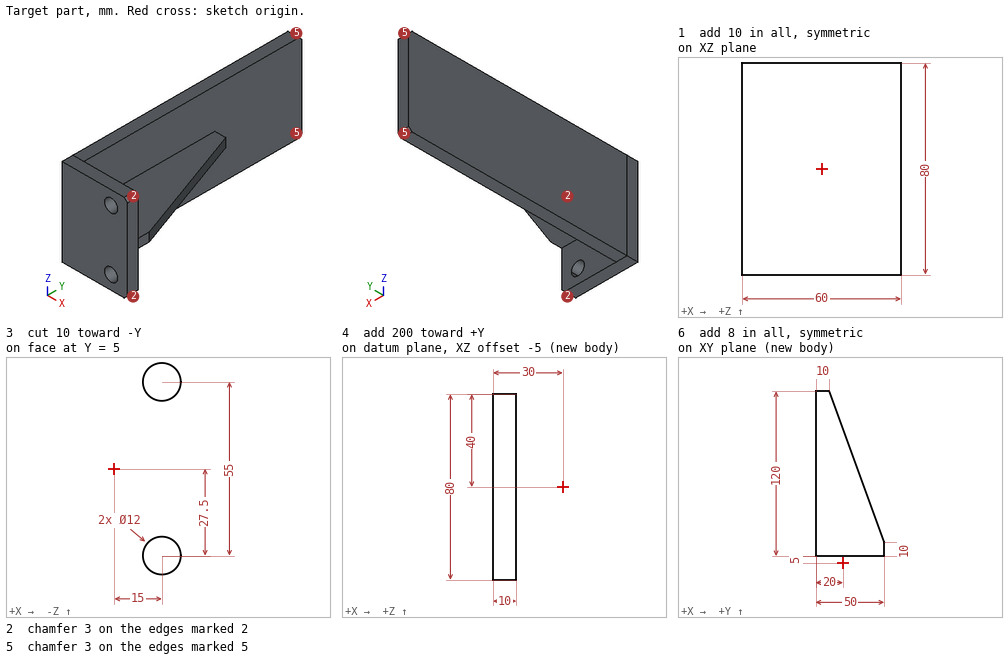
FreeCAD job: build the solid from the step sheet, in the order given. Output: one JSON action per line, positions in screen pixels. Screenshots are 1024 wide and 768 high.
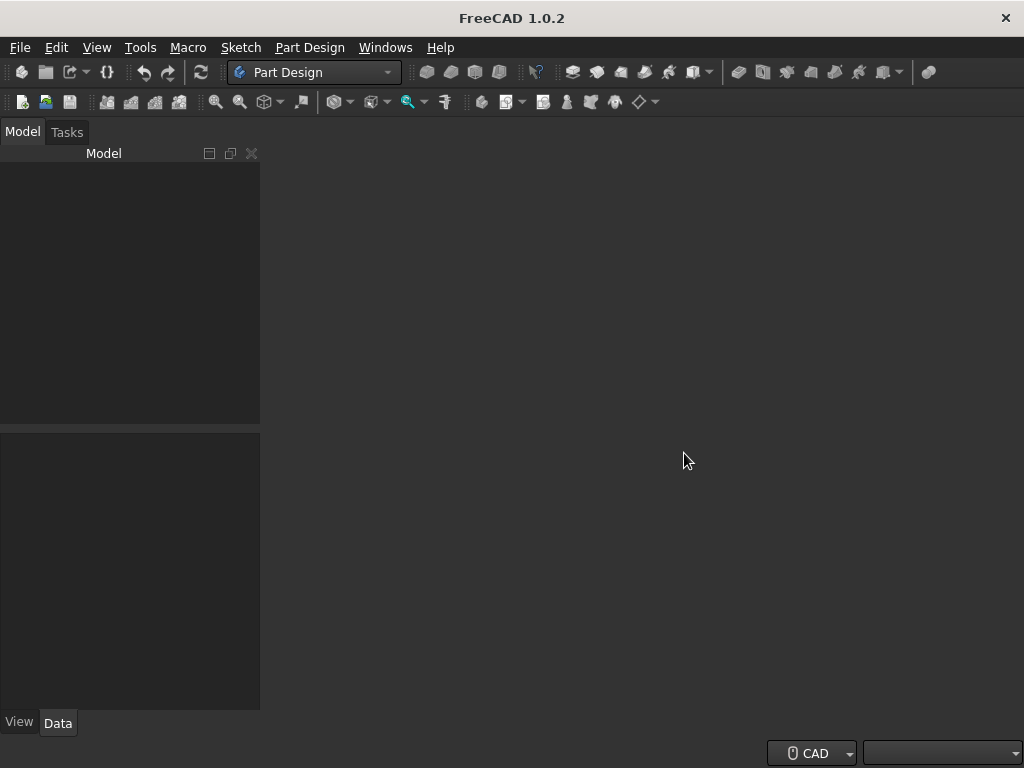
{"action": "left_click", "coordinate": [22, 102]}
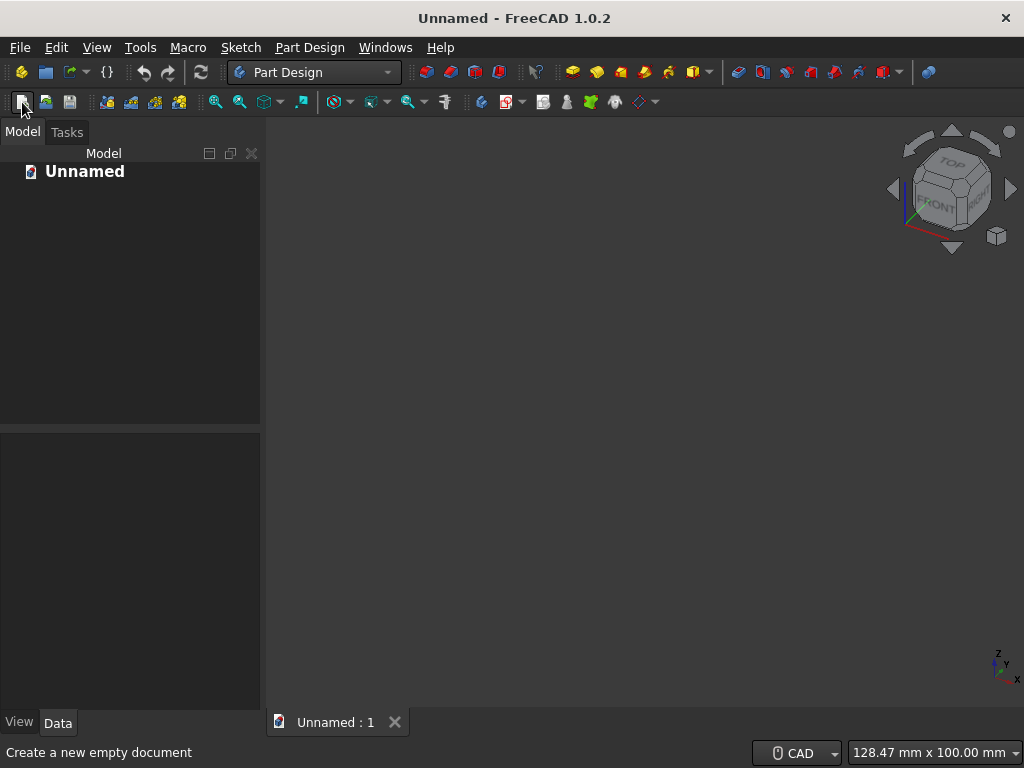
{"action": "left_click", "coordinate": [506, 102]}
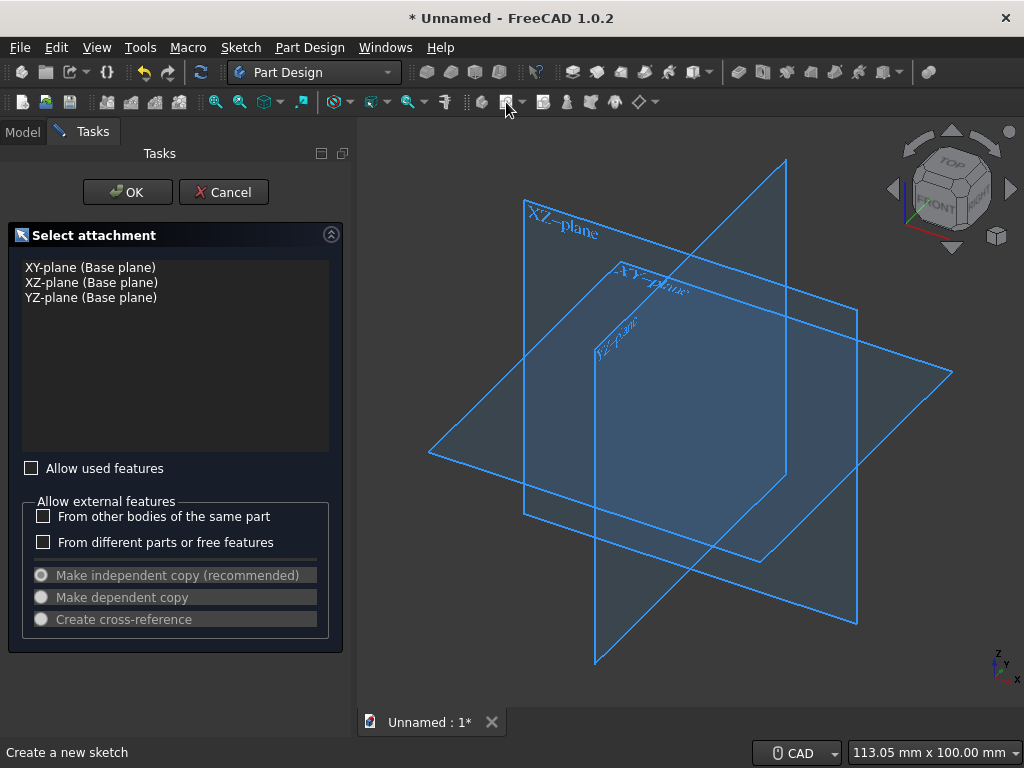
{"action": "left_click", "coordinate": [82, 282]}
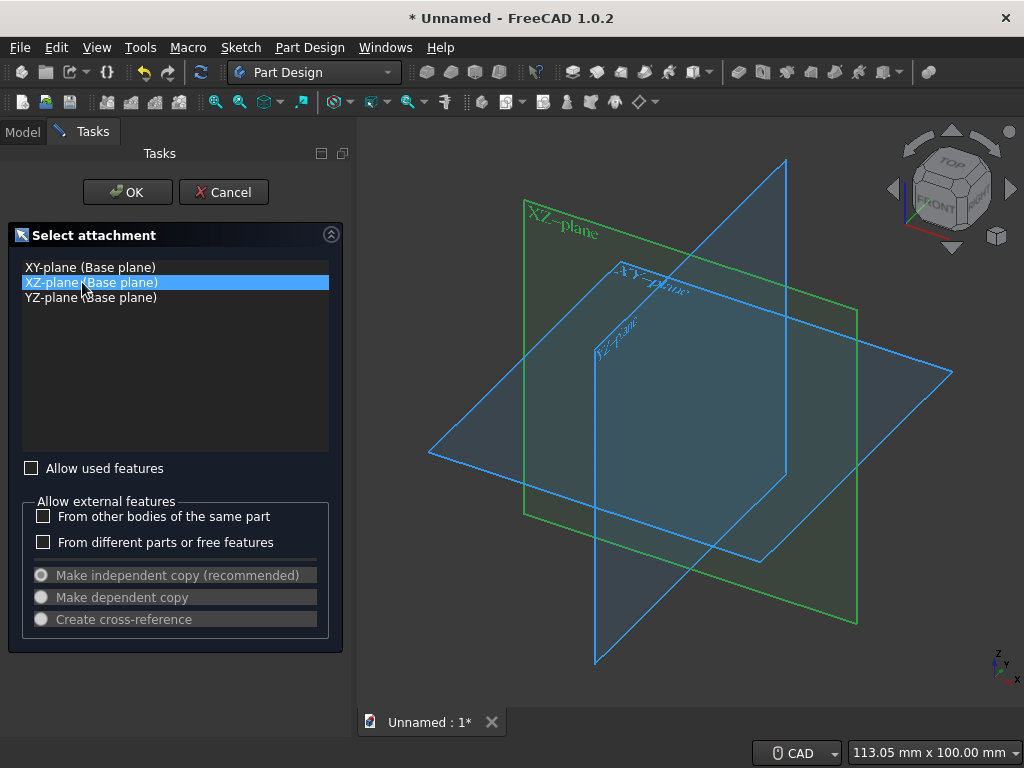
{"action": "left_click", "coordinate": [128, 192]}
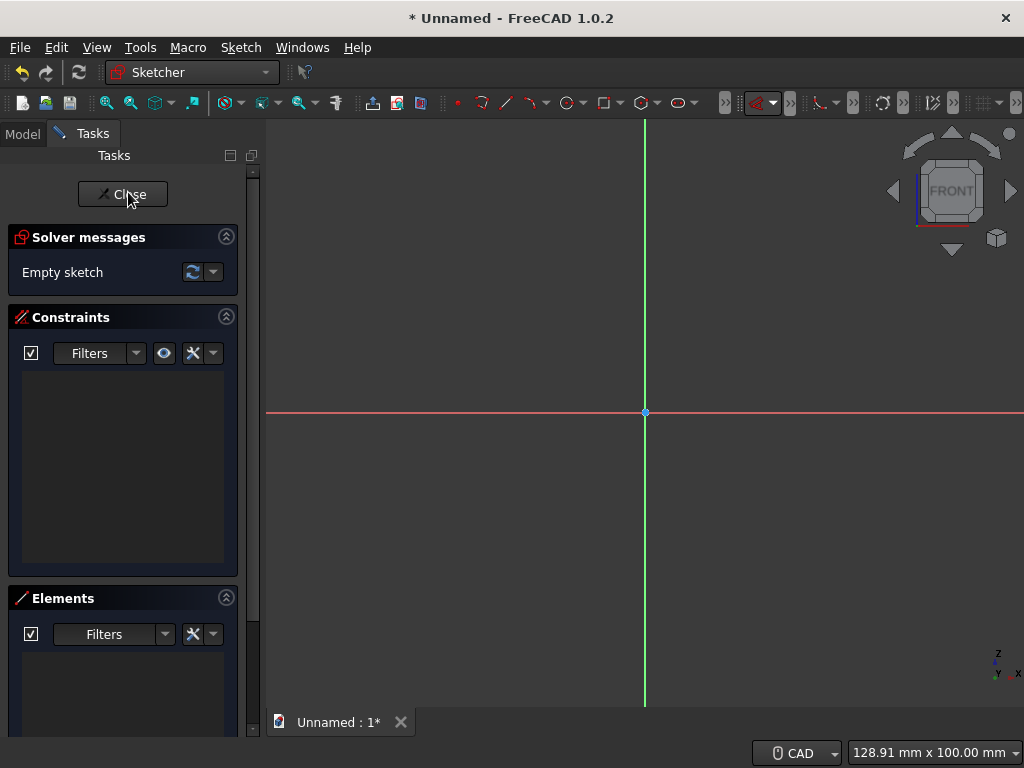
{"action": "key", "text": "g v"}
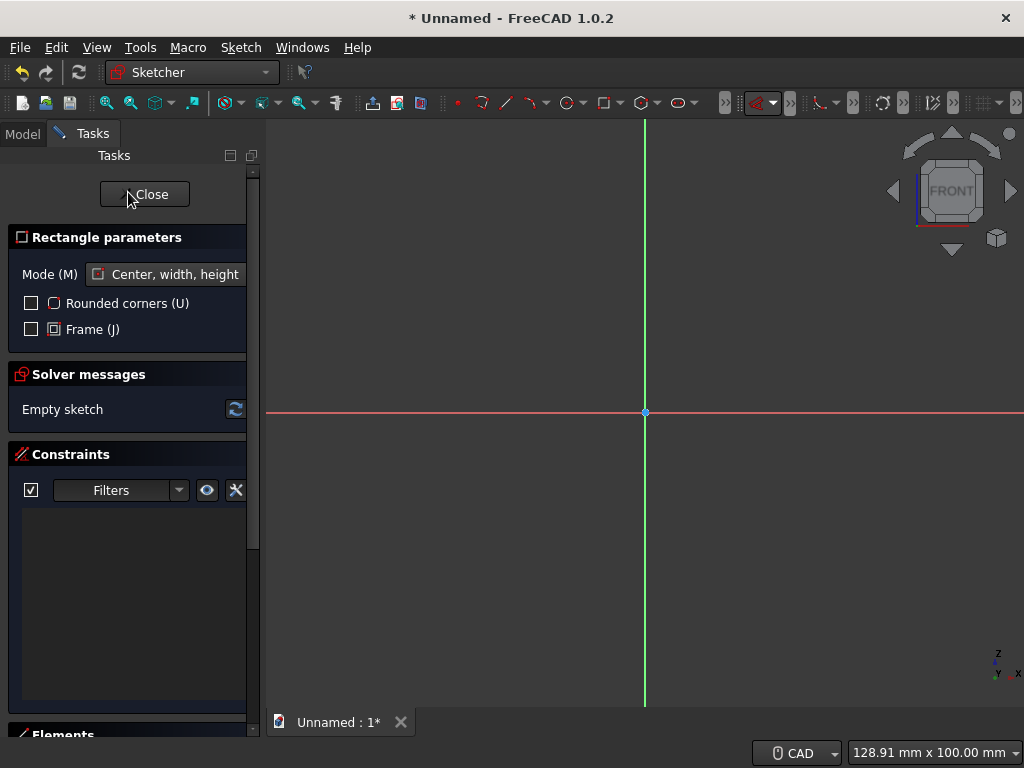
{"action": "left_click", "coordinate": [645, 413]}
{"action": "mouse_move", "coordinate": [821, 178]}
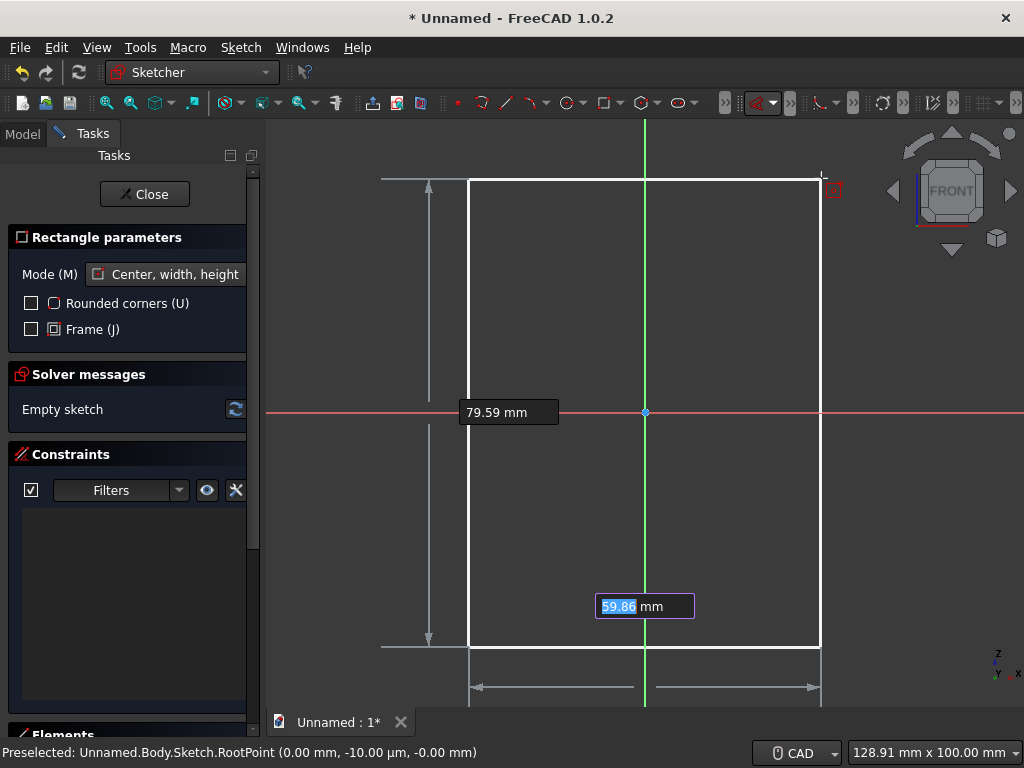
{"action": "type", "text": "60"}
{"action": "key", "text": "Tab"}
{"action": "type", "text": "80"}
{"action": "key", "text": "Return"}
{"action": "key", "text": "Escape"}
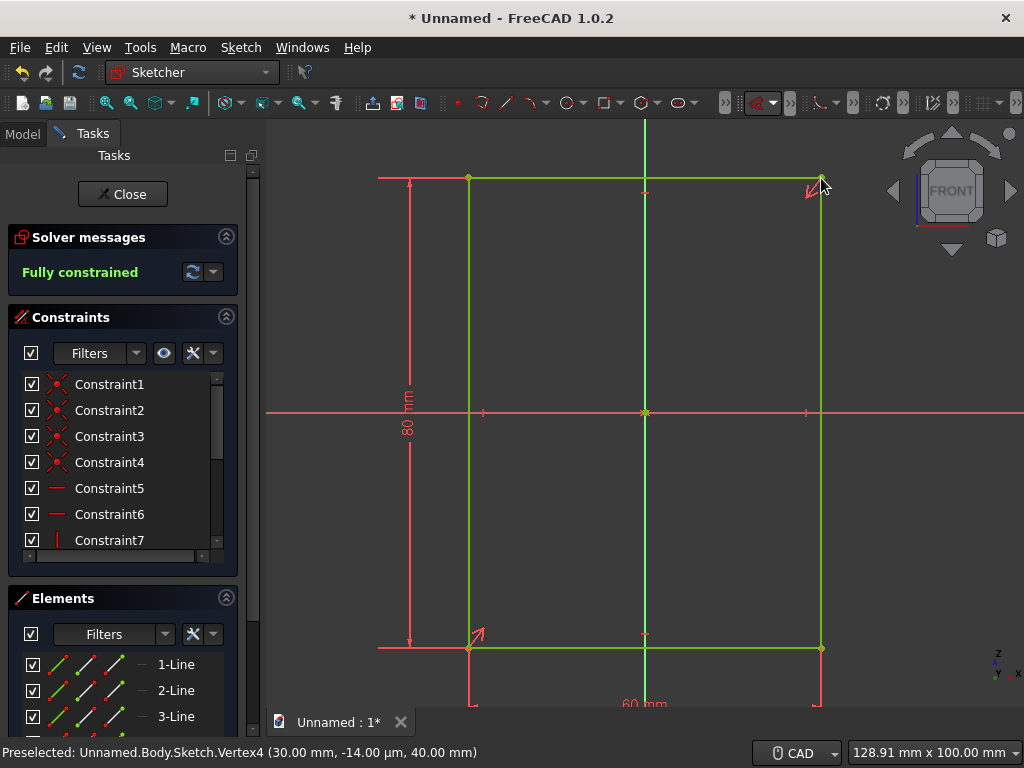
{"action": "left_click", "coordinate": [123, 194]}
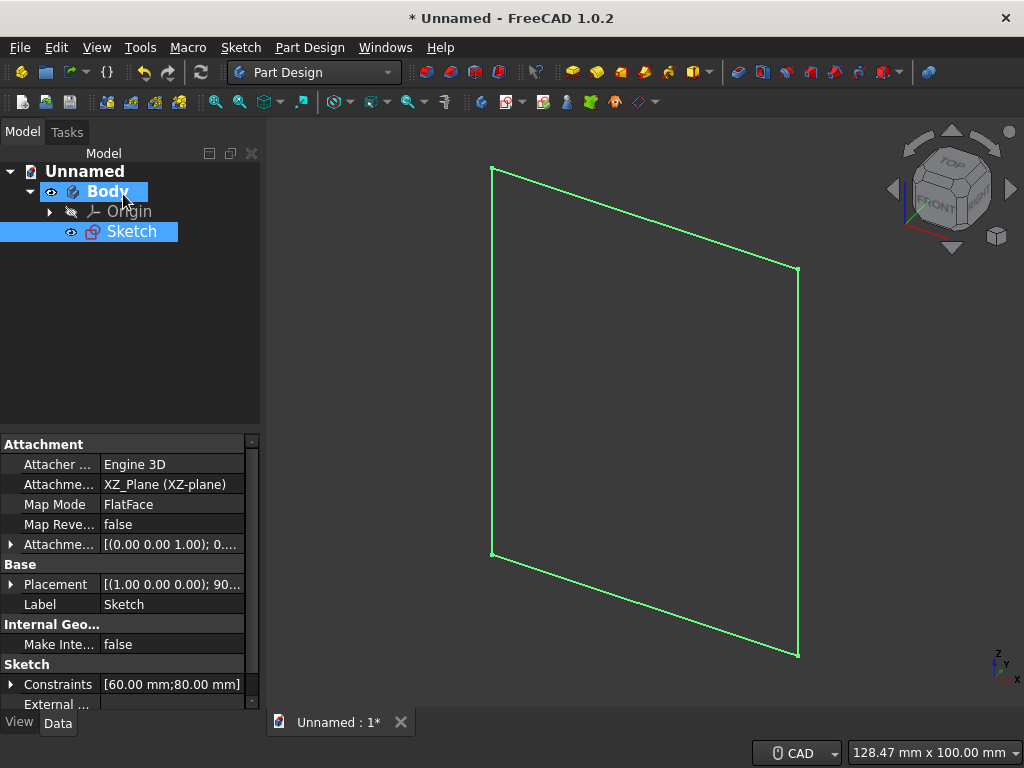
{"action": "left_click", "coordinate": [574, 72]}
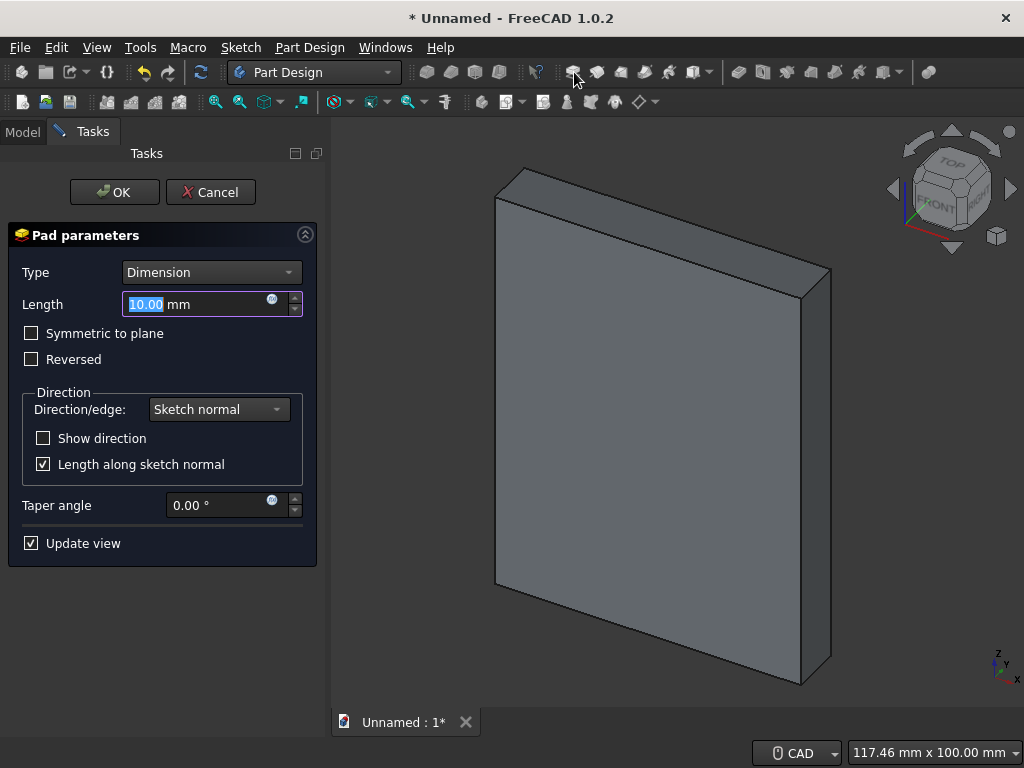
{"action": "type", "text": "10"}
{"action": "key", "text": "Tab"}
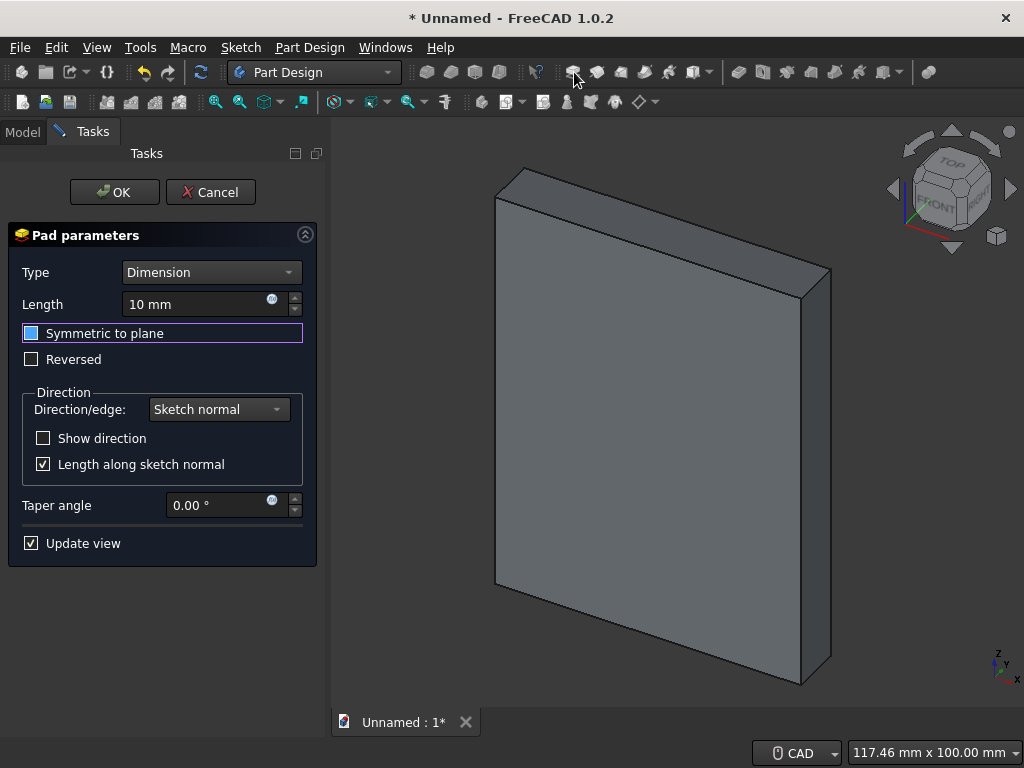
{"action": "left_click", "coordinate": [30, 333]}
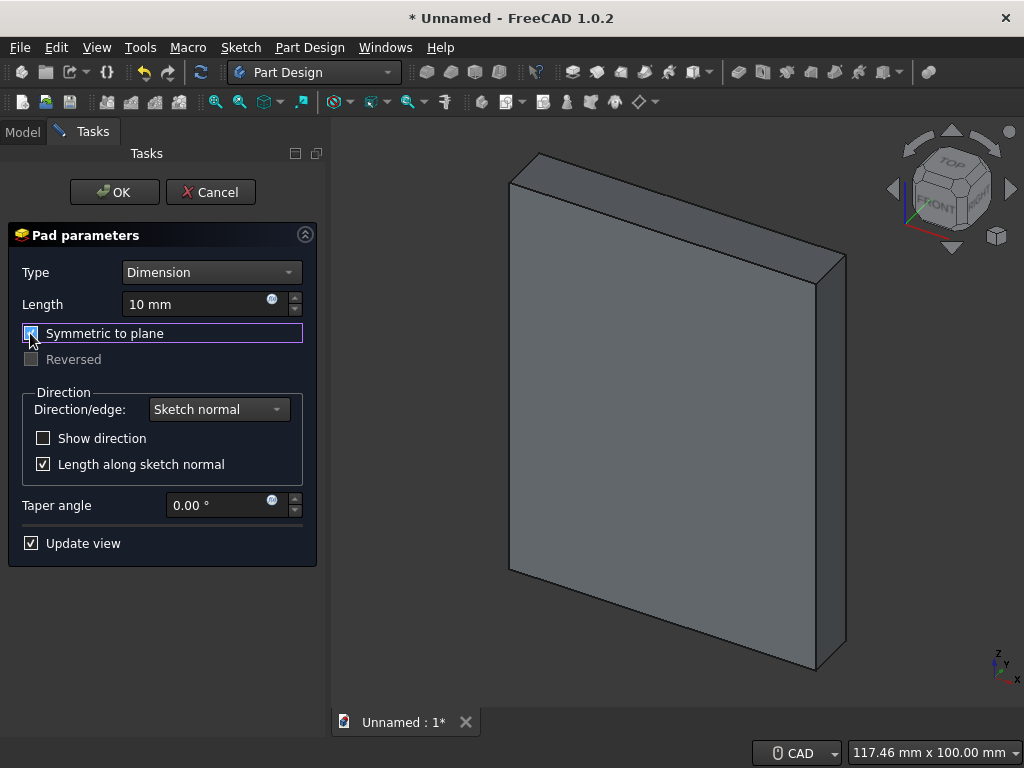
{"action": "left_click", "coordinate": [115, 192]}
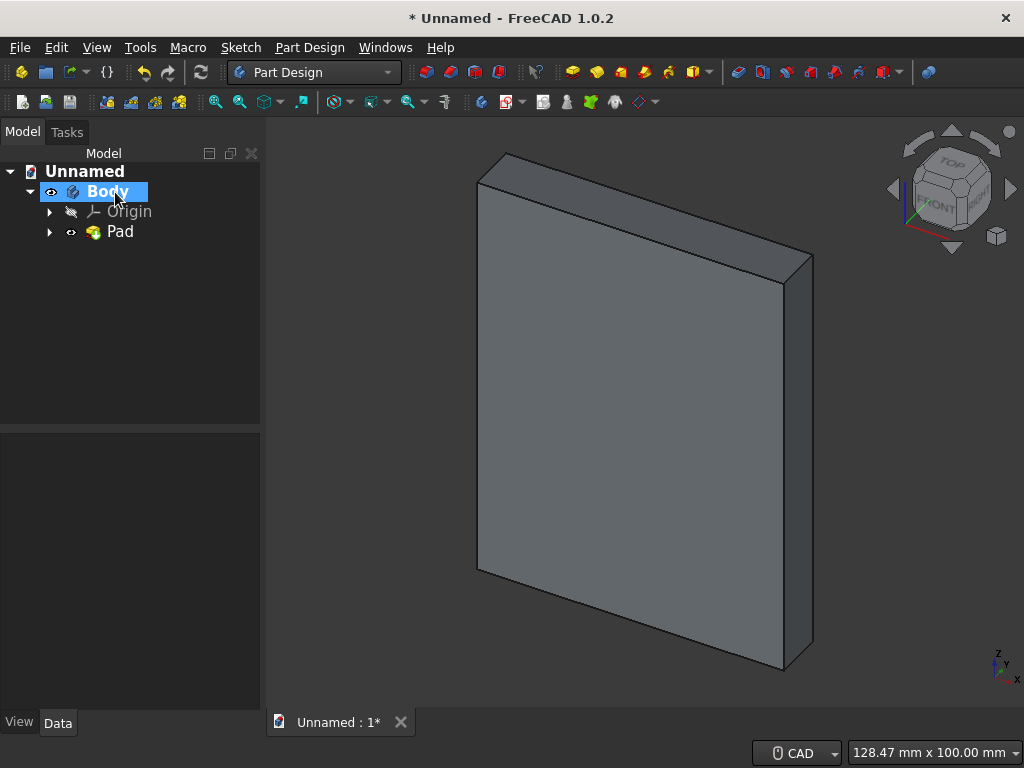
{"action": "left_click", "coordinate": [798, 268]}